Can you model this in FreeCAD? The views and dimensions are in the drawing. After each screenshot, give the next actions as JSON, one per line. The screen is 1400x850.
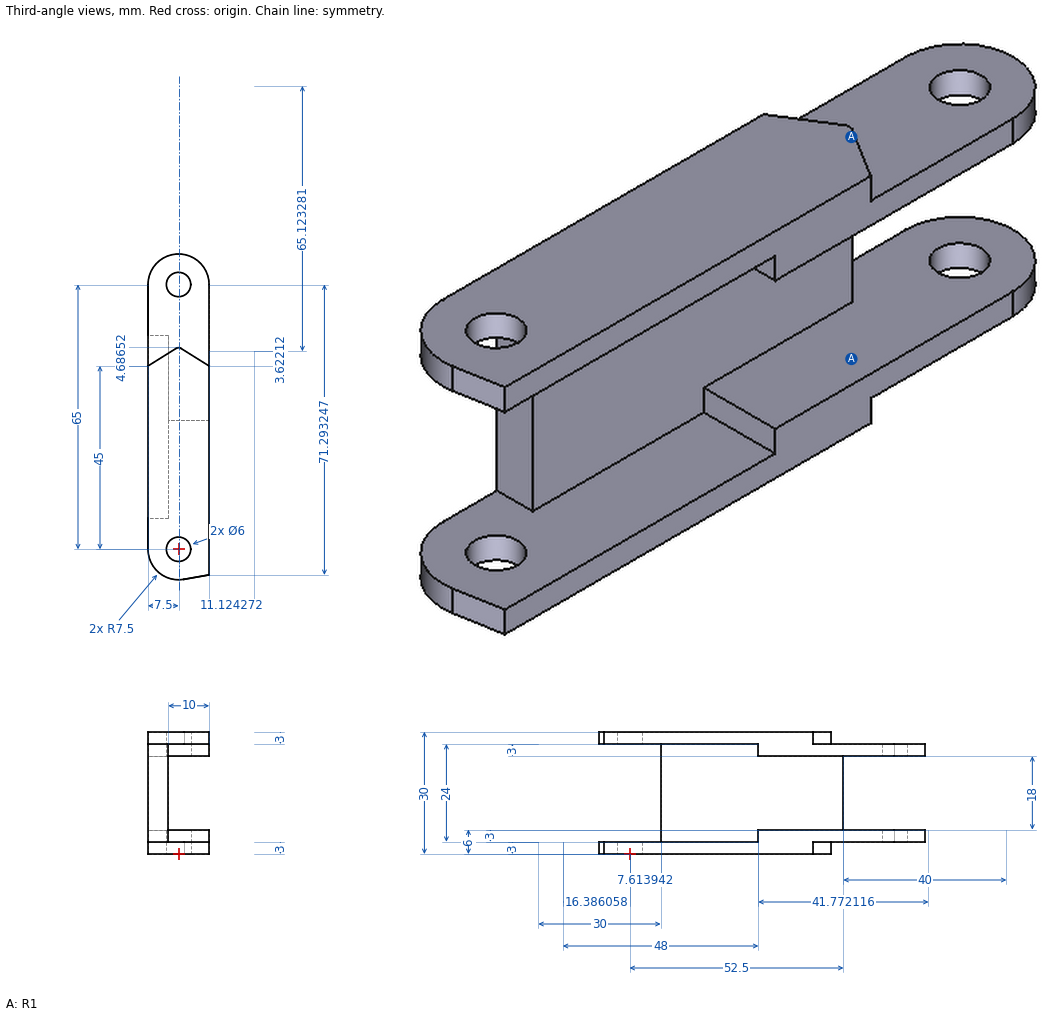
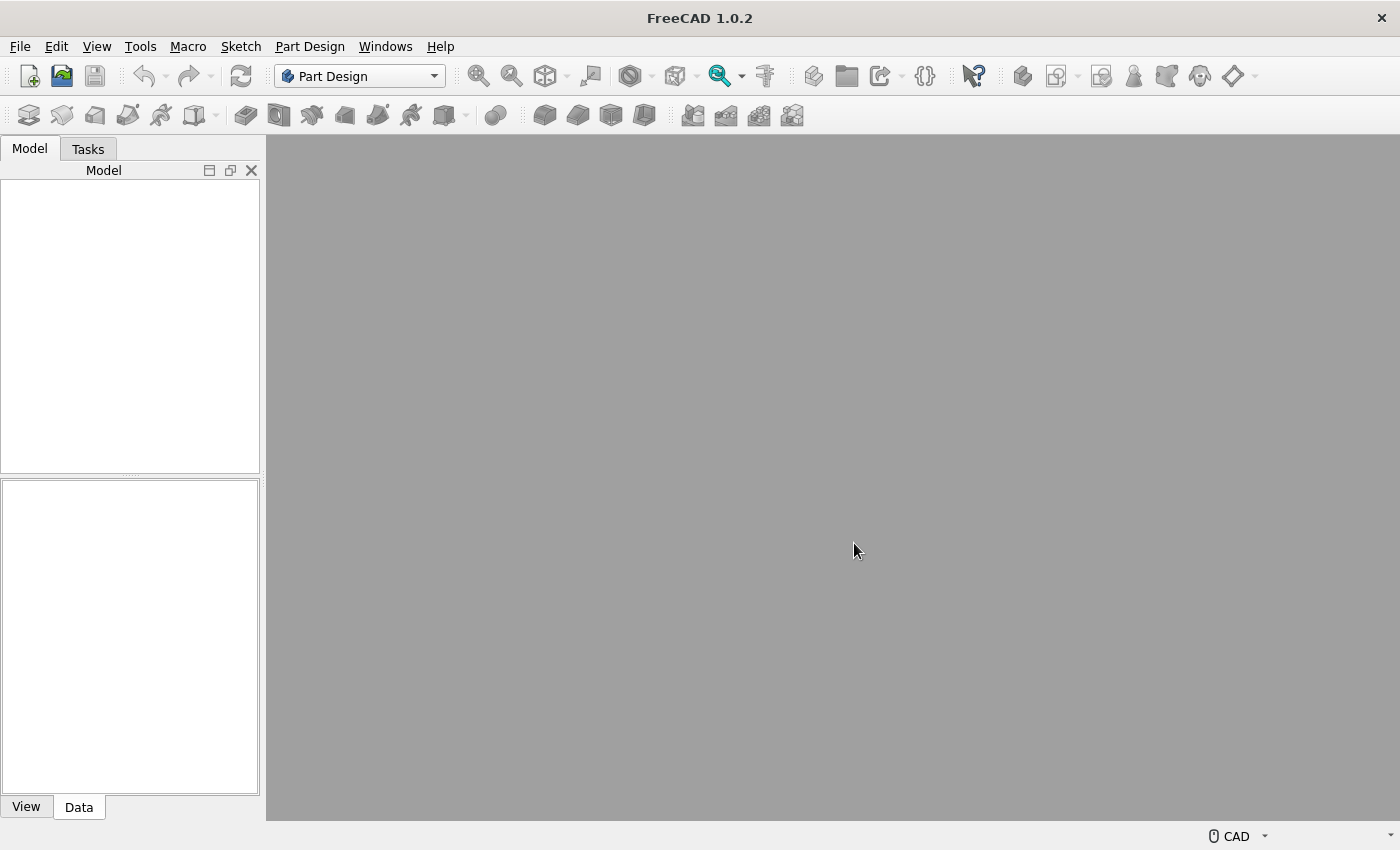
{"action": "key", "text": "ctrl+n"}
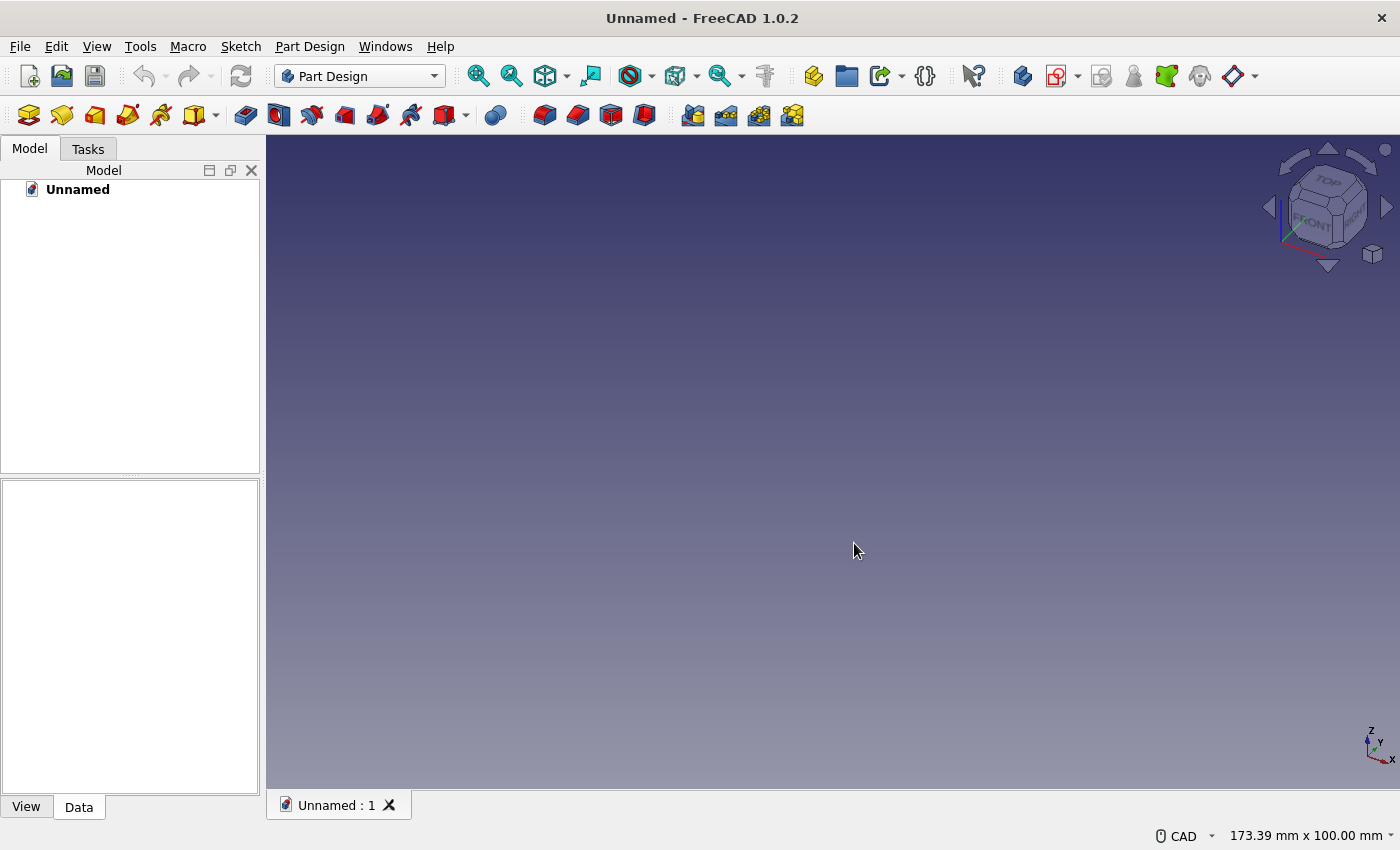
{"action": "left_click", "coordinate": [1056, 76]}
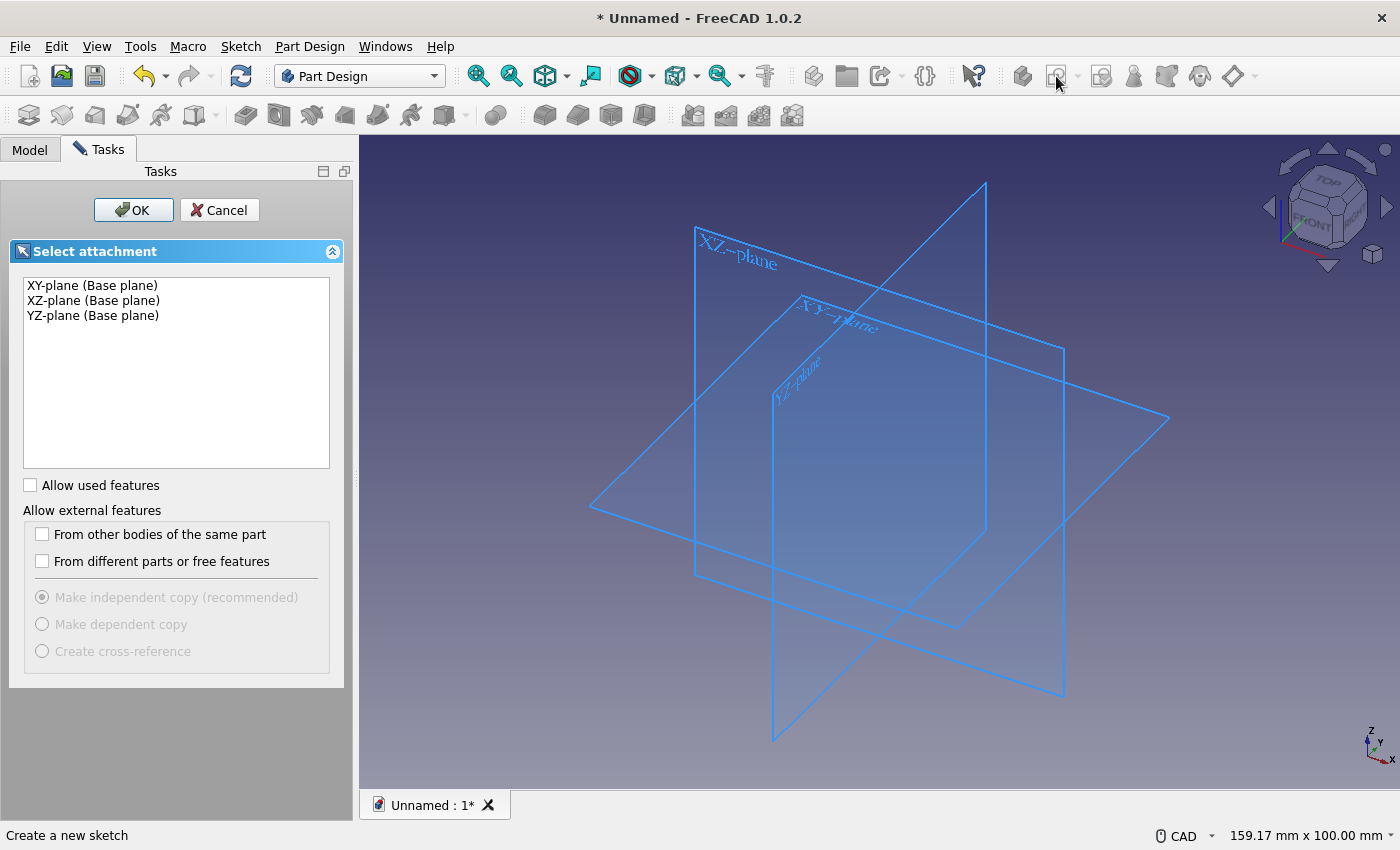
{"action": "left_click", "coordinate": [84, 286]}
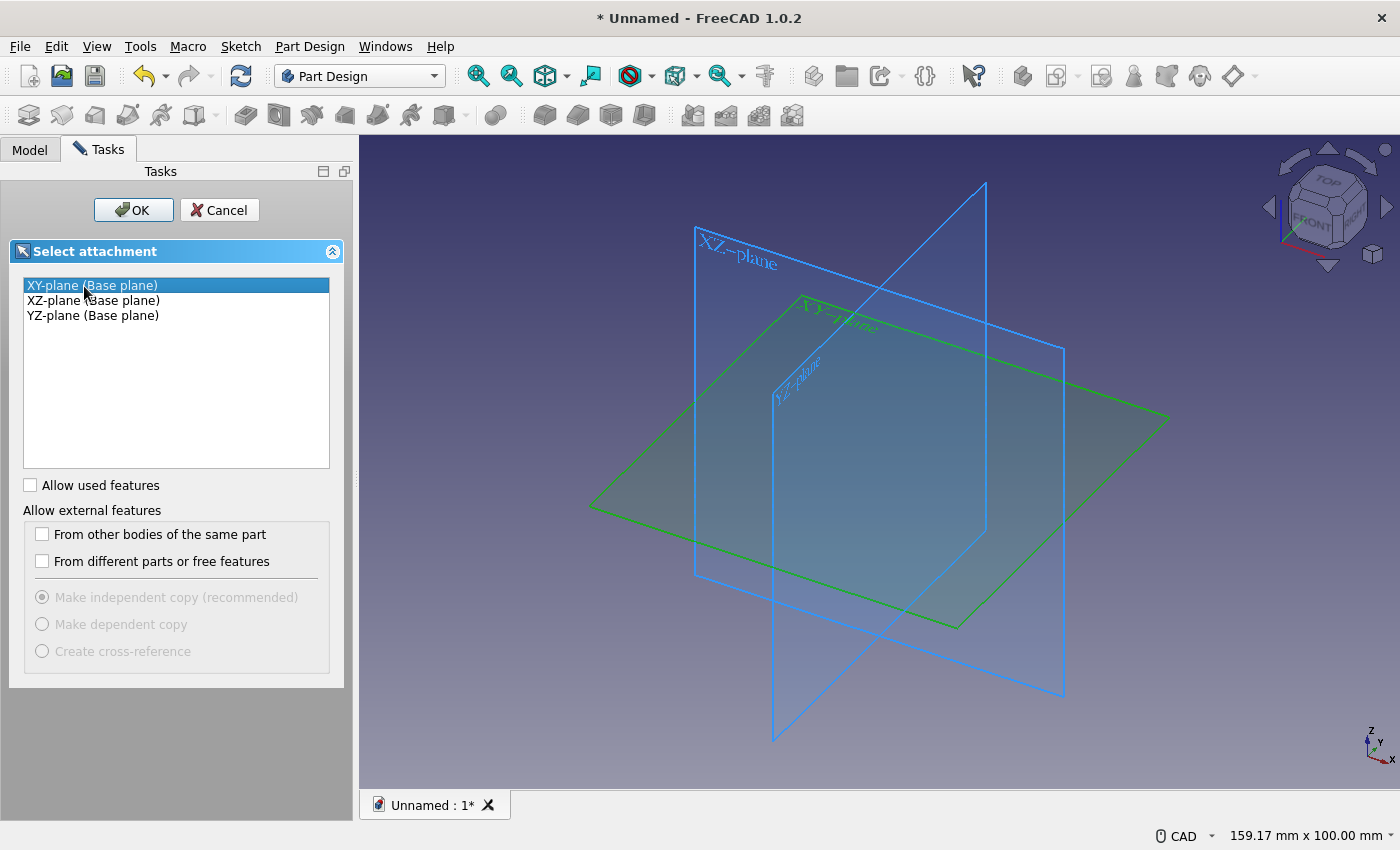
{"action": "left_click", "coordinate": [134, 210]}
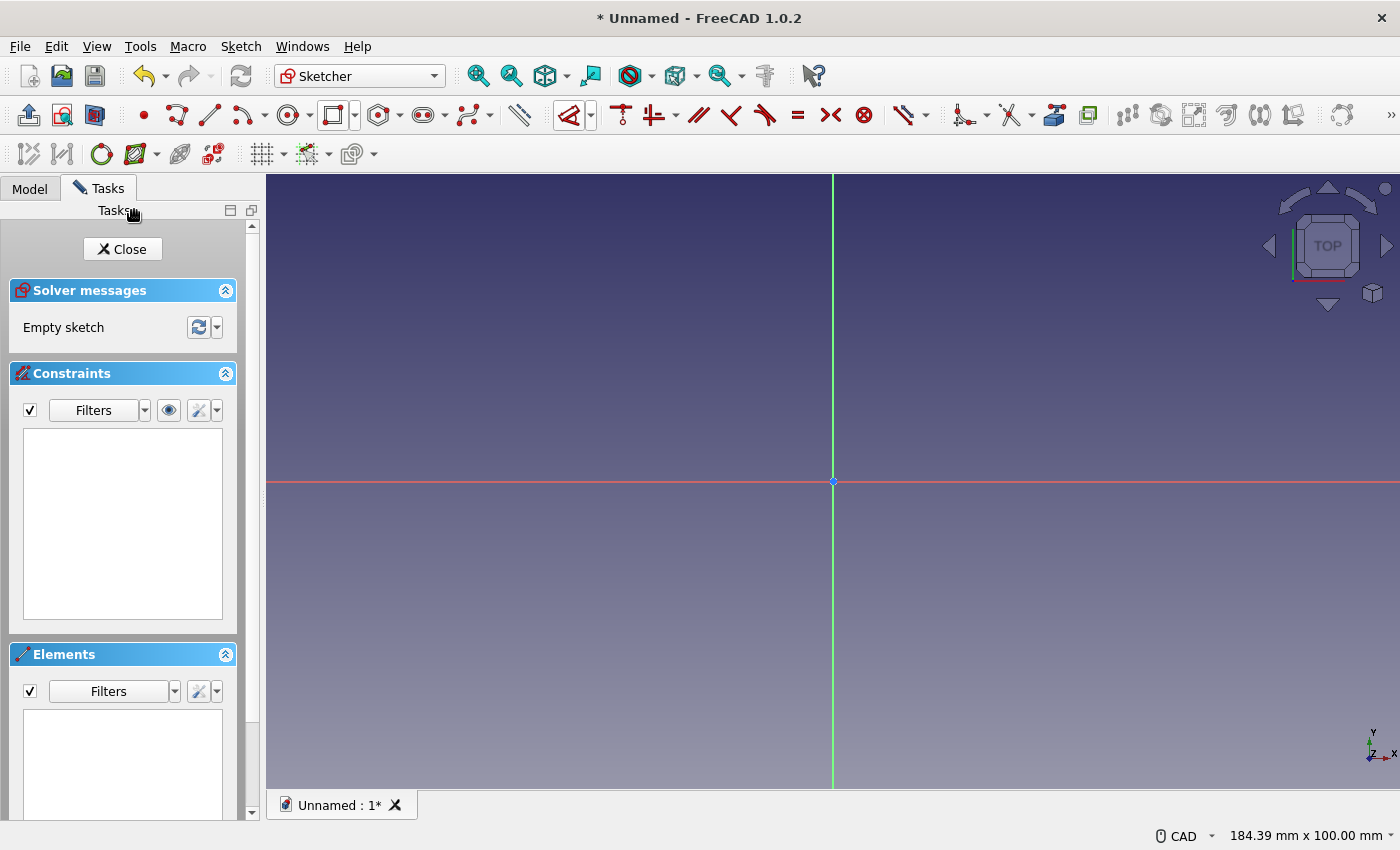
{"action": "scroll", "coordinate": [625, 761], "scroll_direction": "down", "scroll_amount": 2}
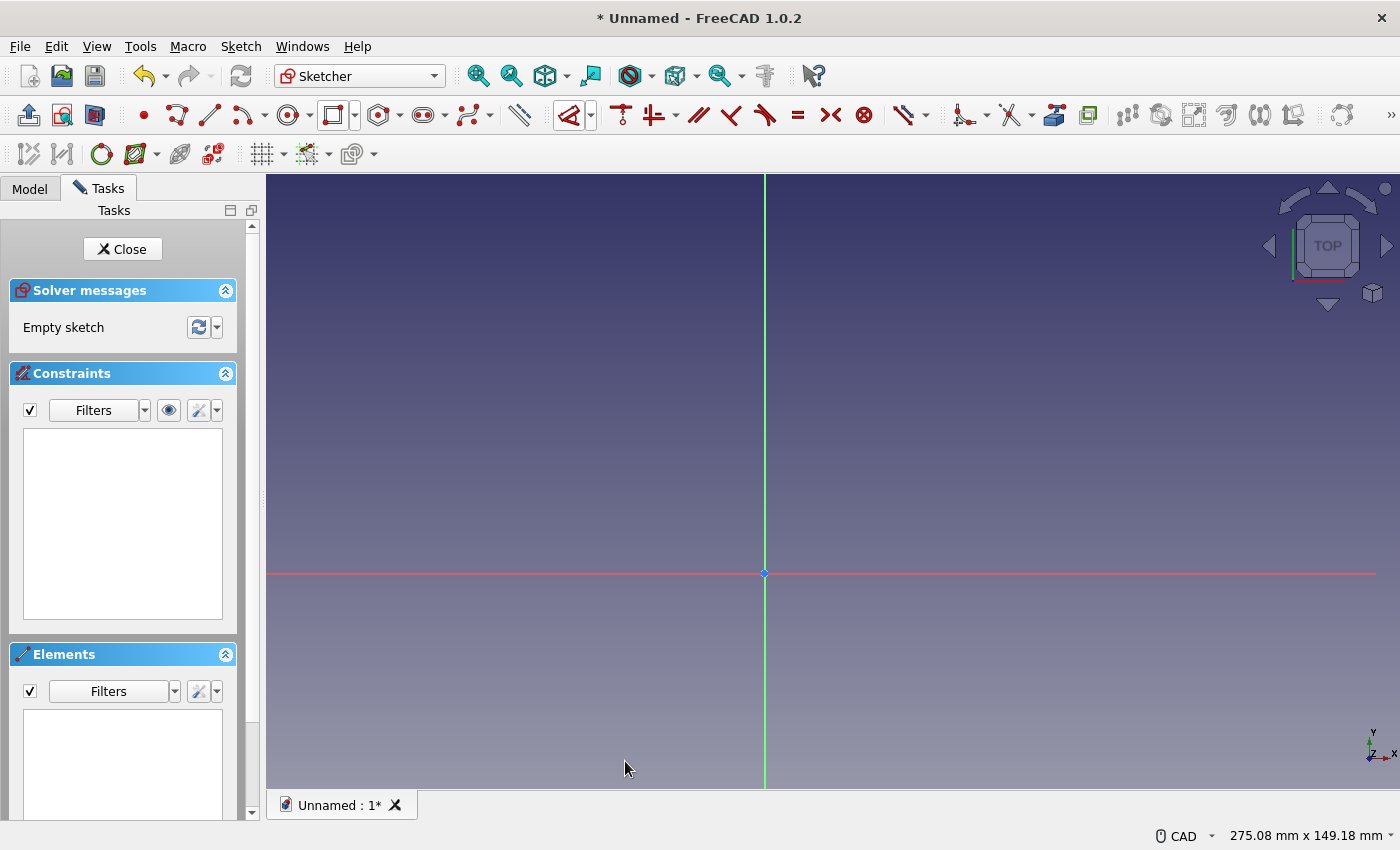
{"action": "left_click", "coordinate": [210, 116]}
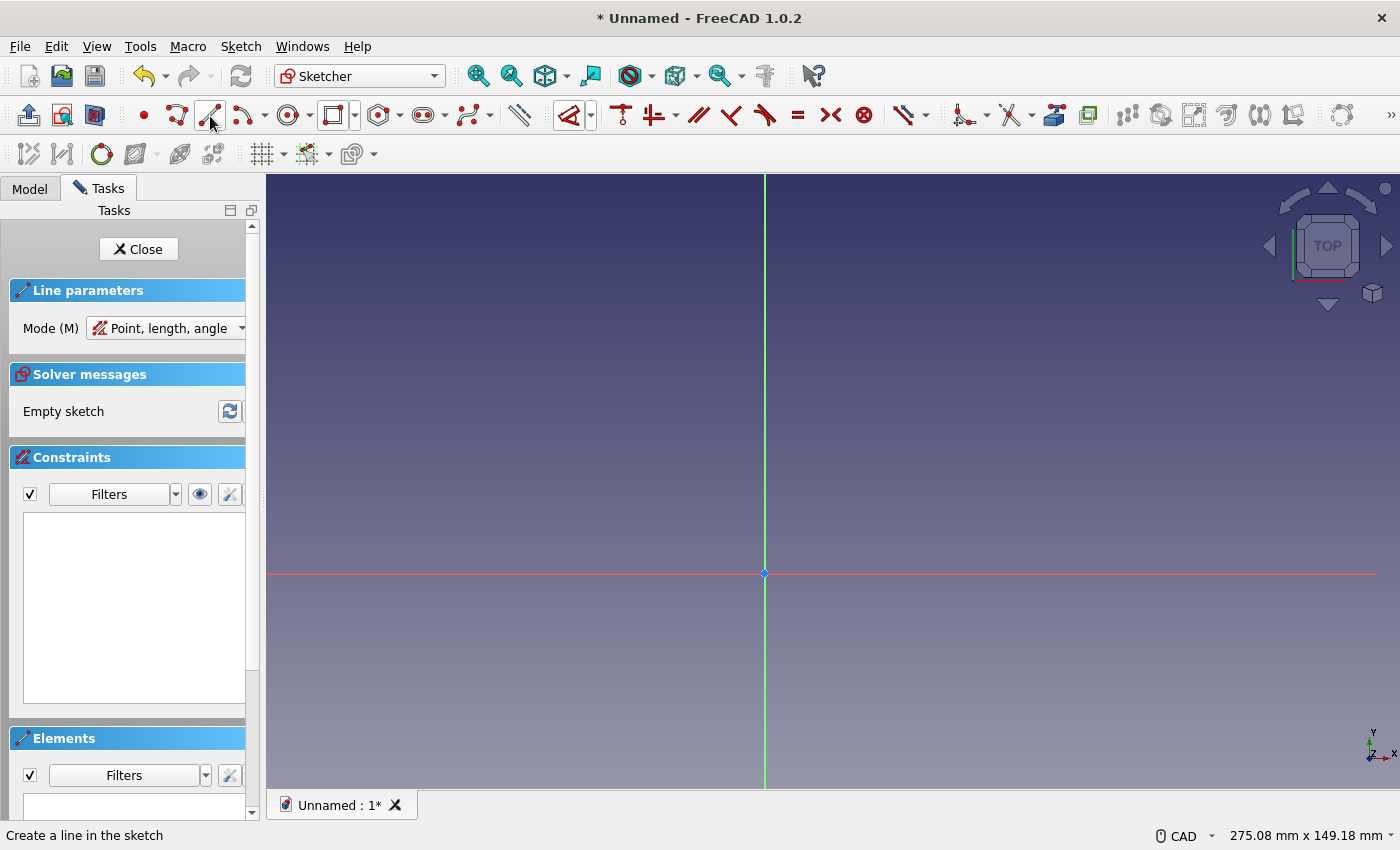
{"action": "left_click", "coordinate": [734, 306]}
{"action": "left_click", "coordinate": [734, 574]}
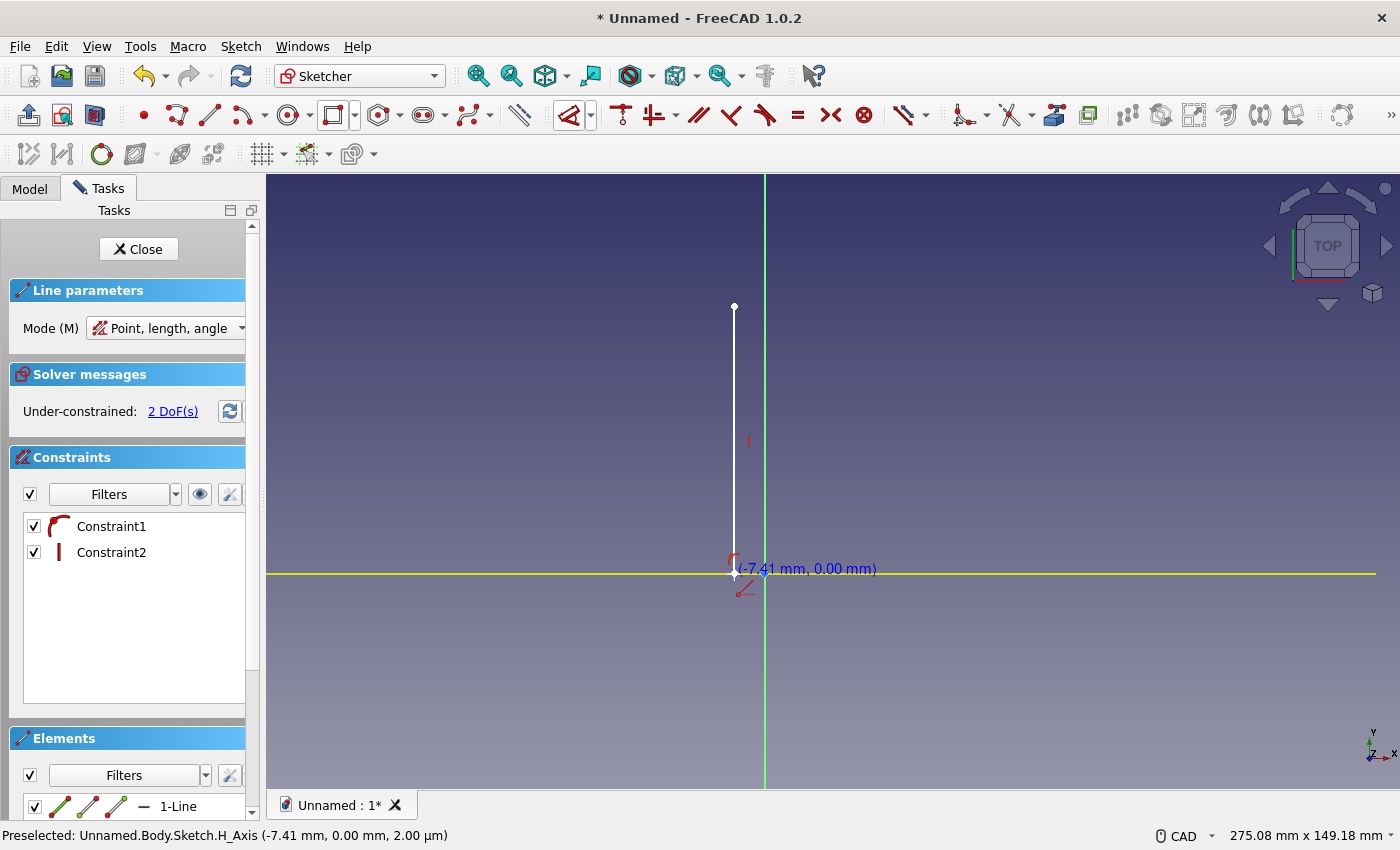
{"action": "left_click", "coordinate": [177, 116]}